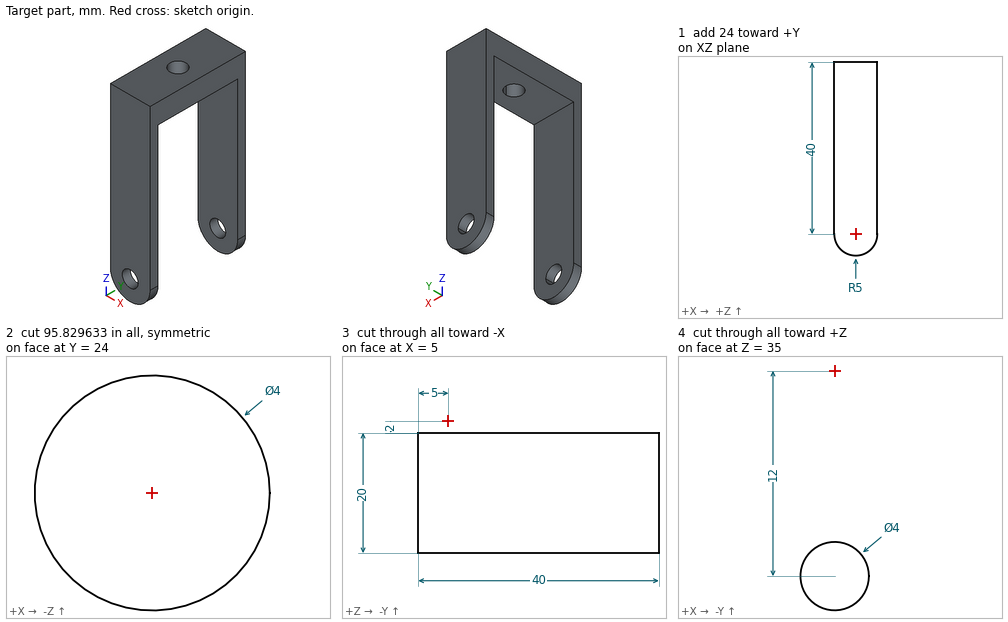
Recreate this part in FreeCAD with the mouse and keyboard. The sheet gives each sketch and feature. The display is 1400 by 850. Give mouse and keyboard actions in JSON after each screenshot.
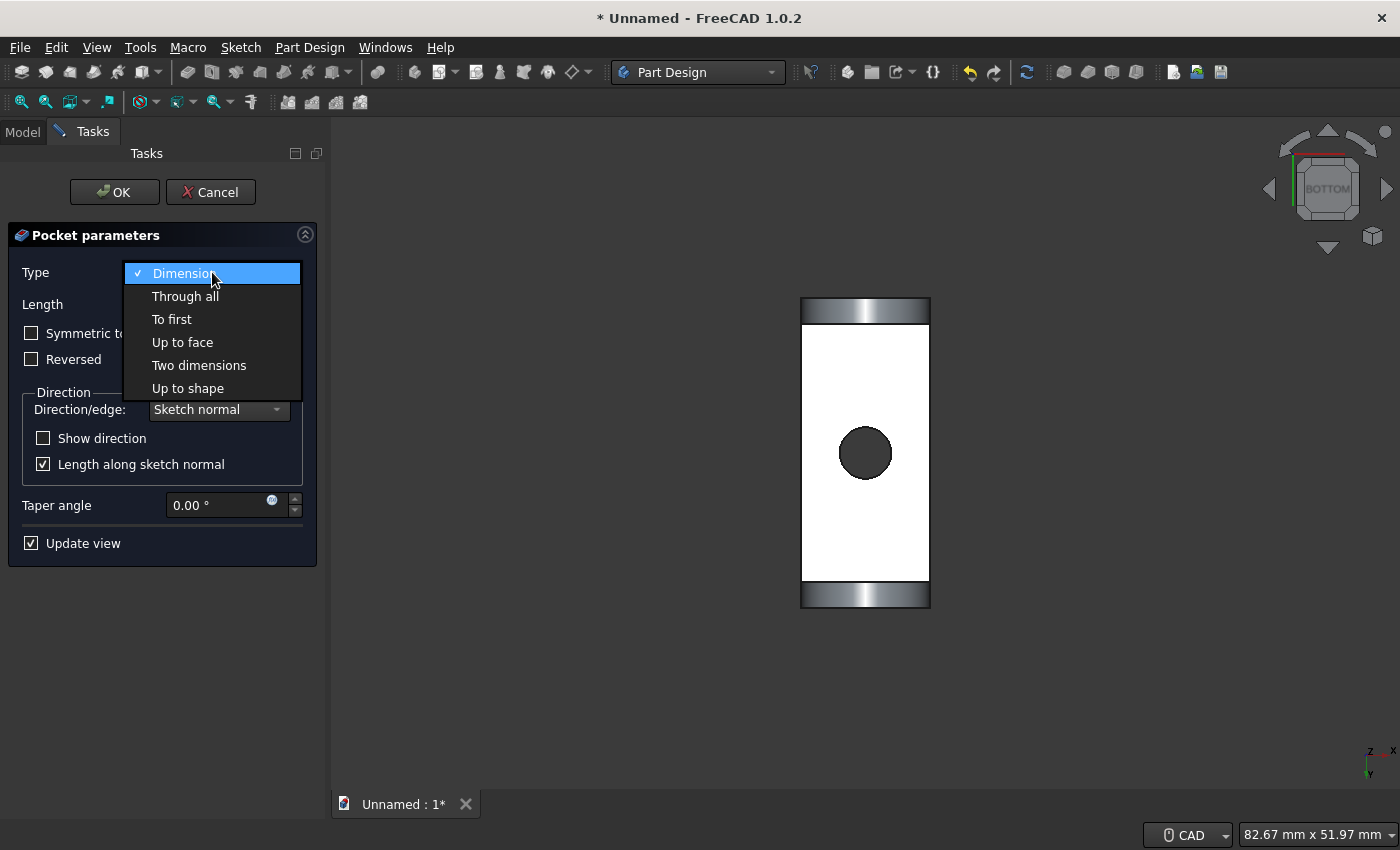
{"action": "left_click", "coordinate": [212, 296]}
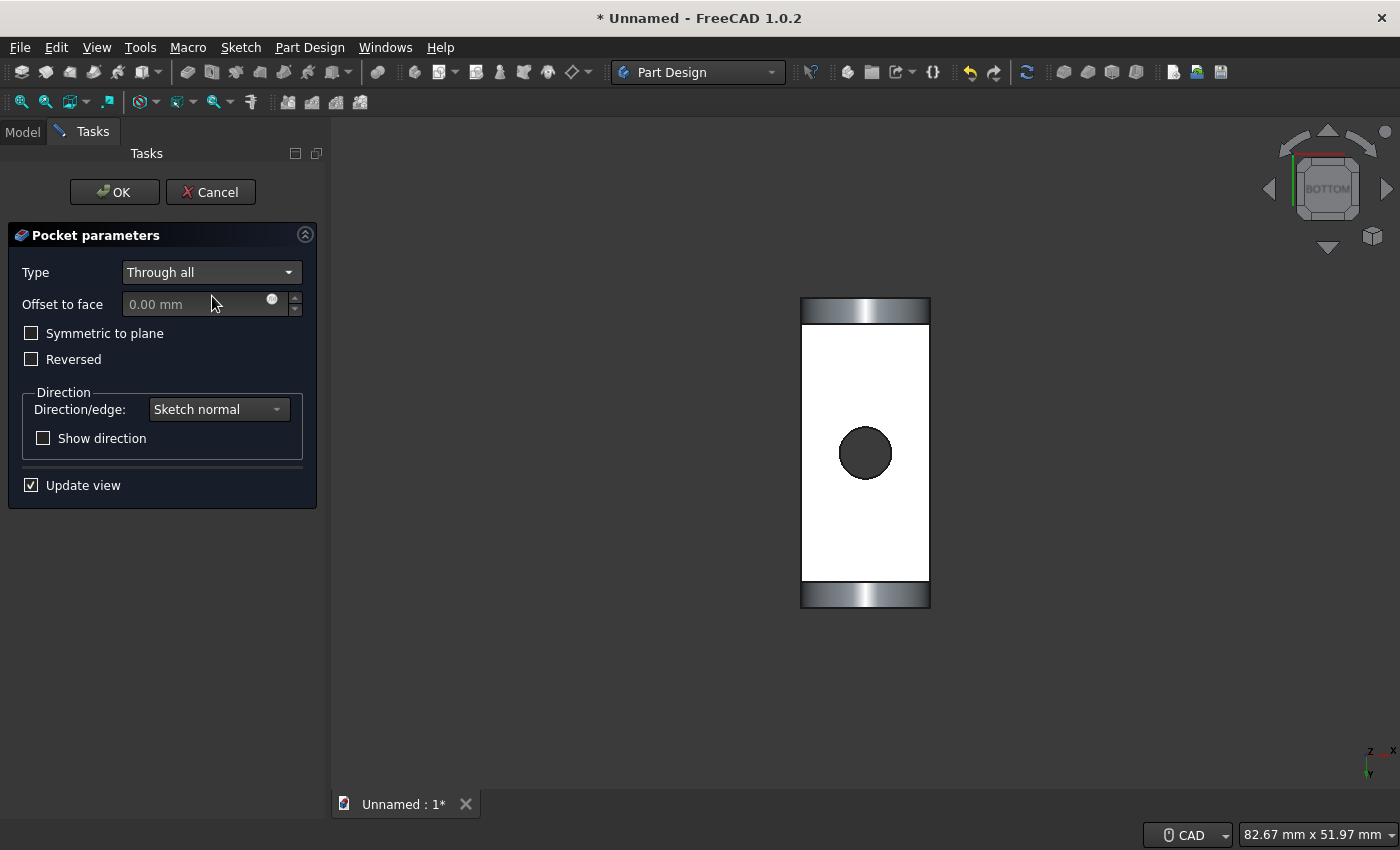
{"action": "left_click", "coordinate": [115, 192]}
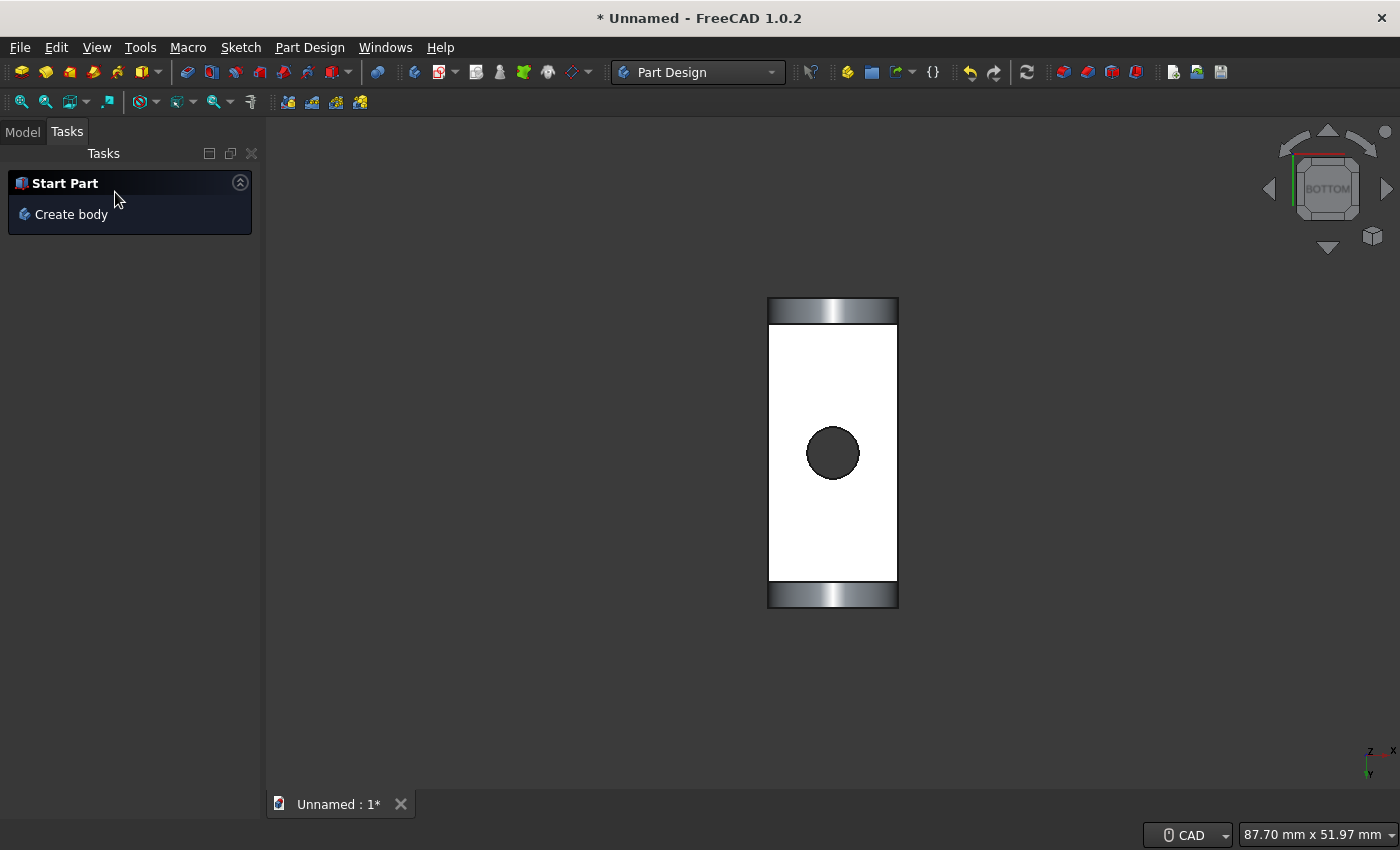
{"action": "key", "text": "0"}